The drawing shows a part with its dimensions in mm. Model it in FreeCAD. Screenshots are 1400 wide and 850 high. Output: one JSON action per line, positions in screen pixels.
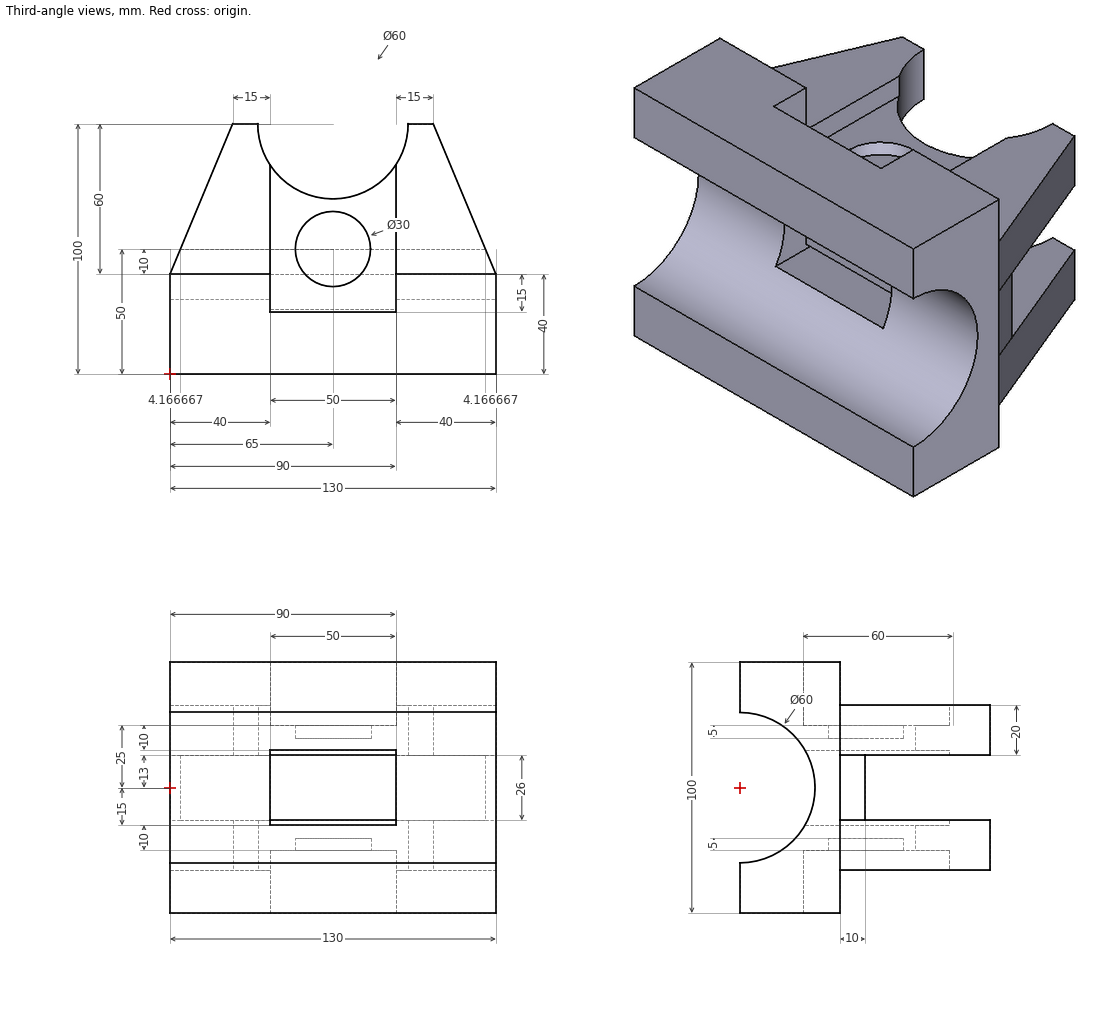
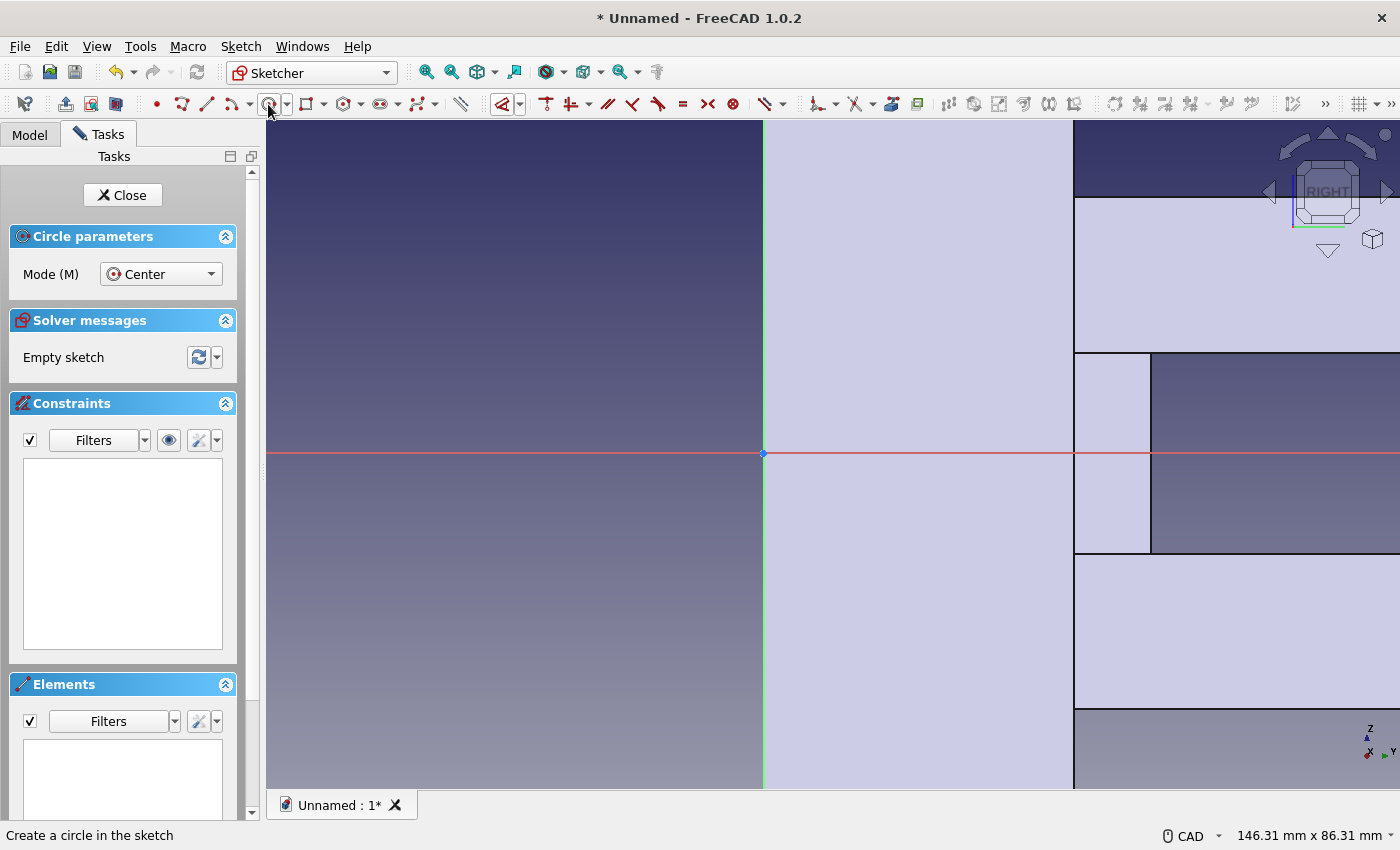
{"action": "left_click", "coordinate": [764, 453]}
{"action": "mouse_move", "coordinate": [928, 289]}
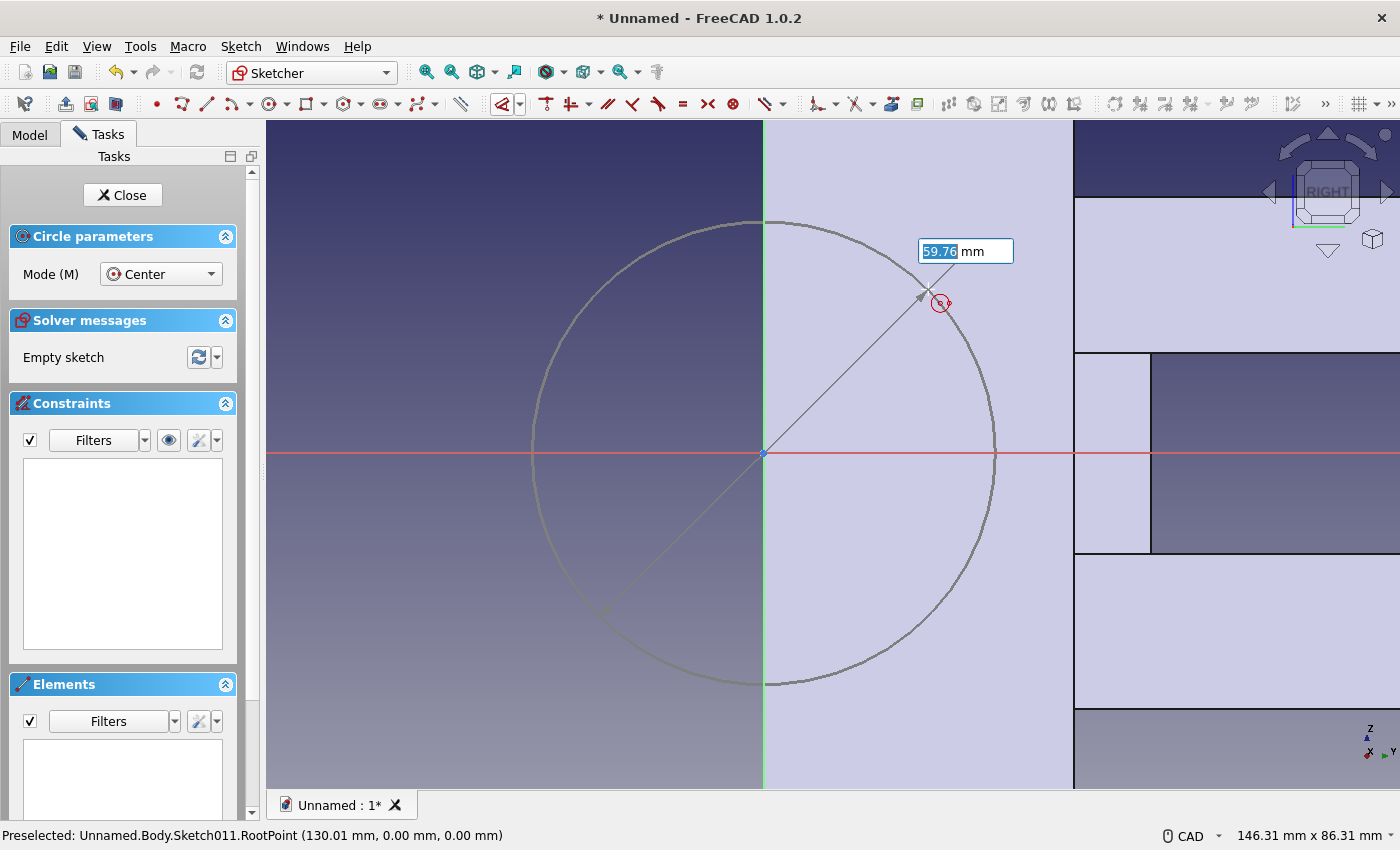
{"action": "type", "text": "60"}
{"action": "key", "text": "Return"}
{"action": "key", "text": "Escape"}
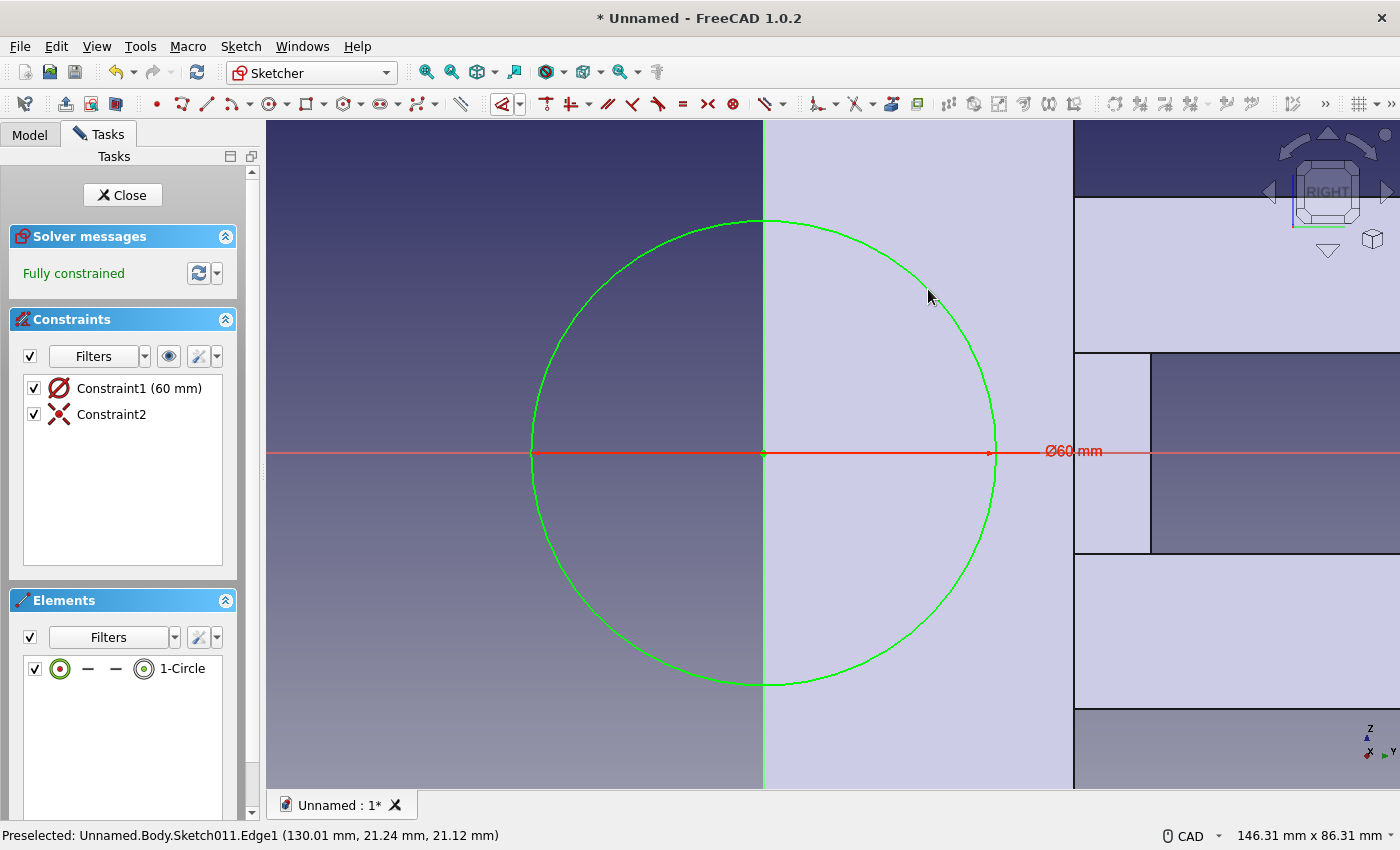
{"action": "left_click", "coordinate": [123, 195]}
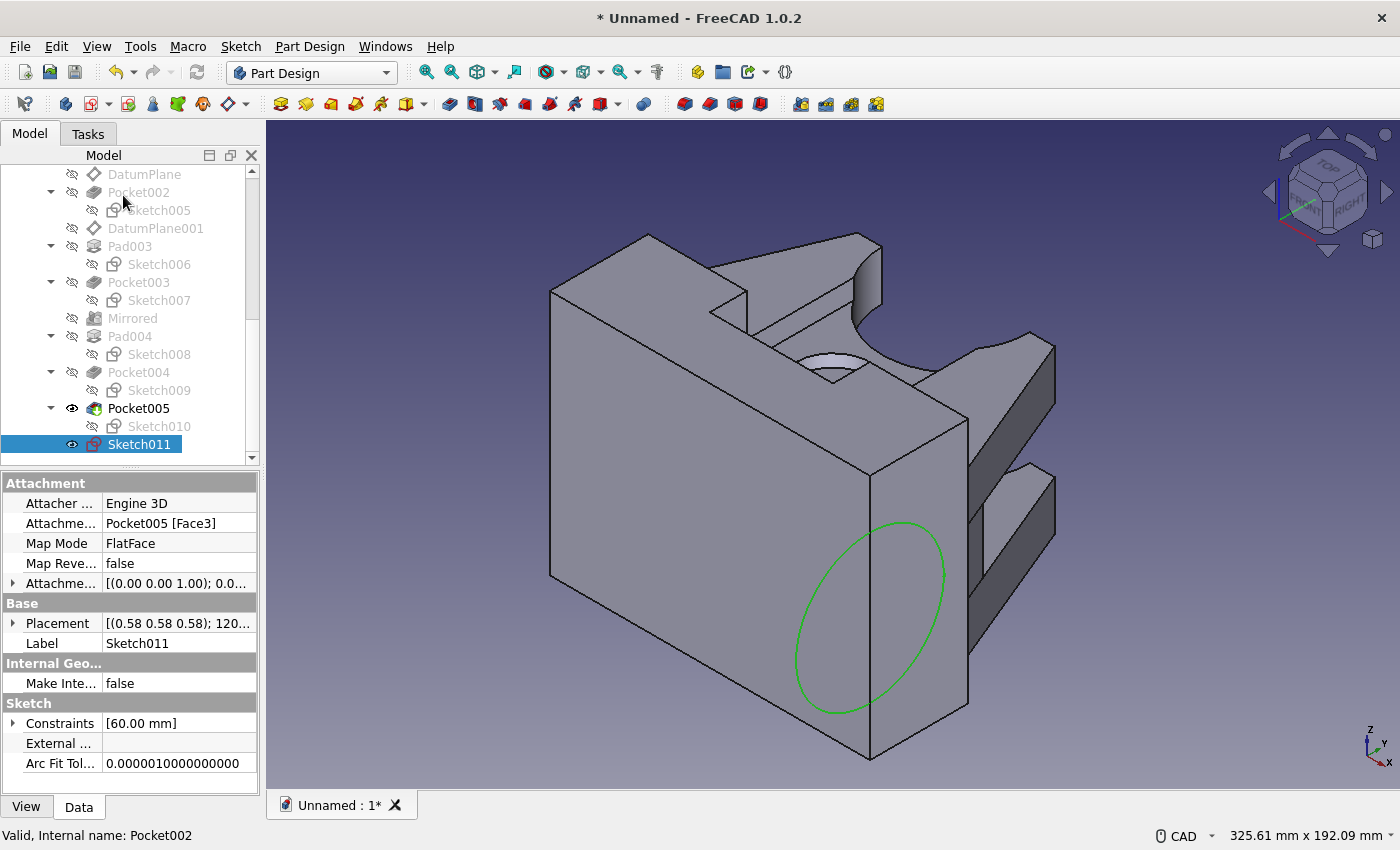
{"action": "left_click", "coordinate": [450, 104]}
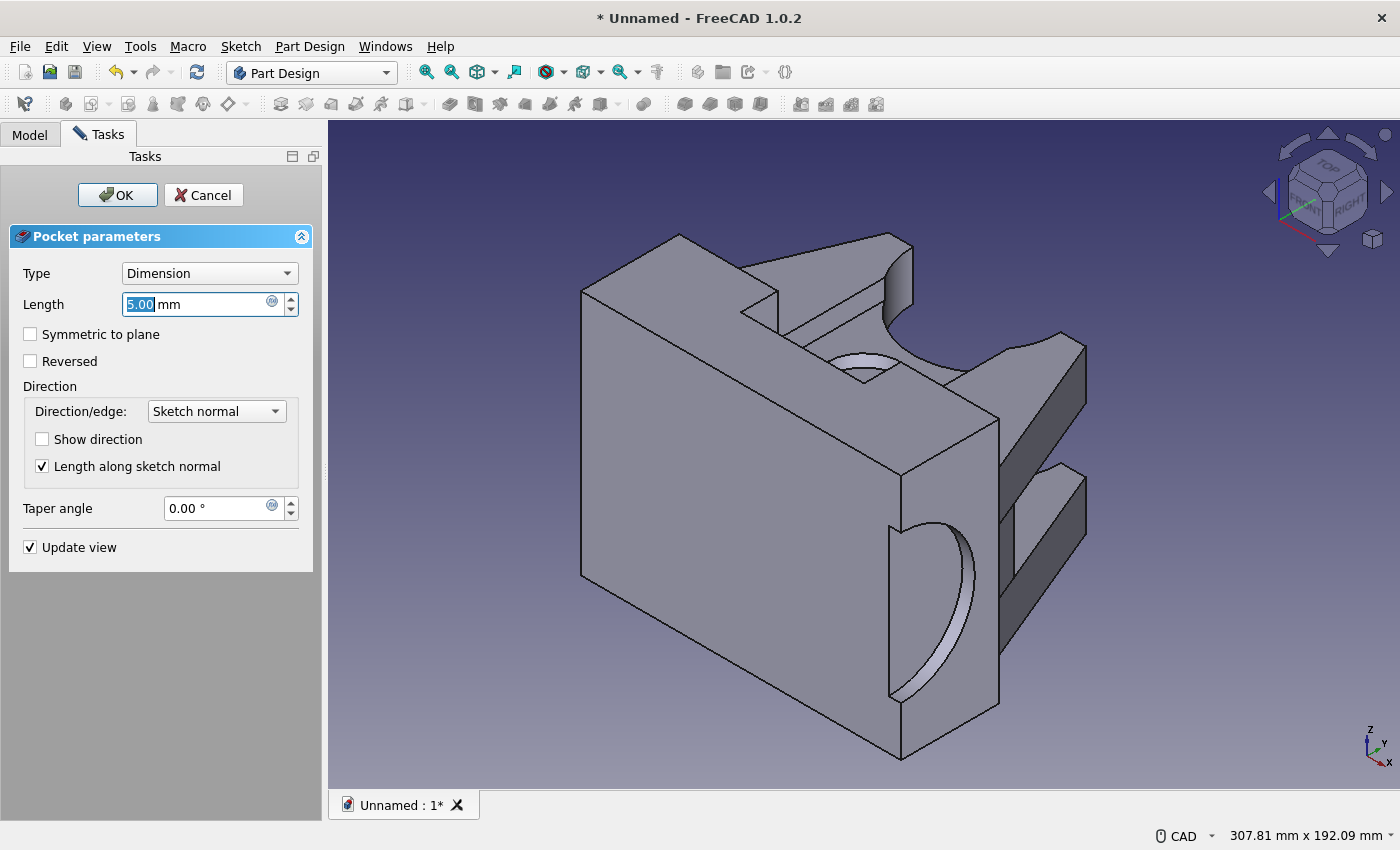
{"action": "left_click", "coordinate": [210, 274]}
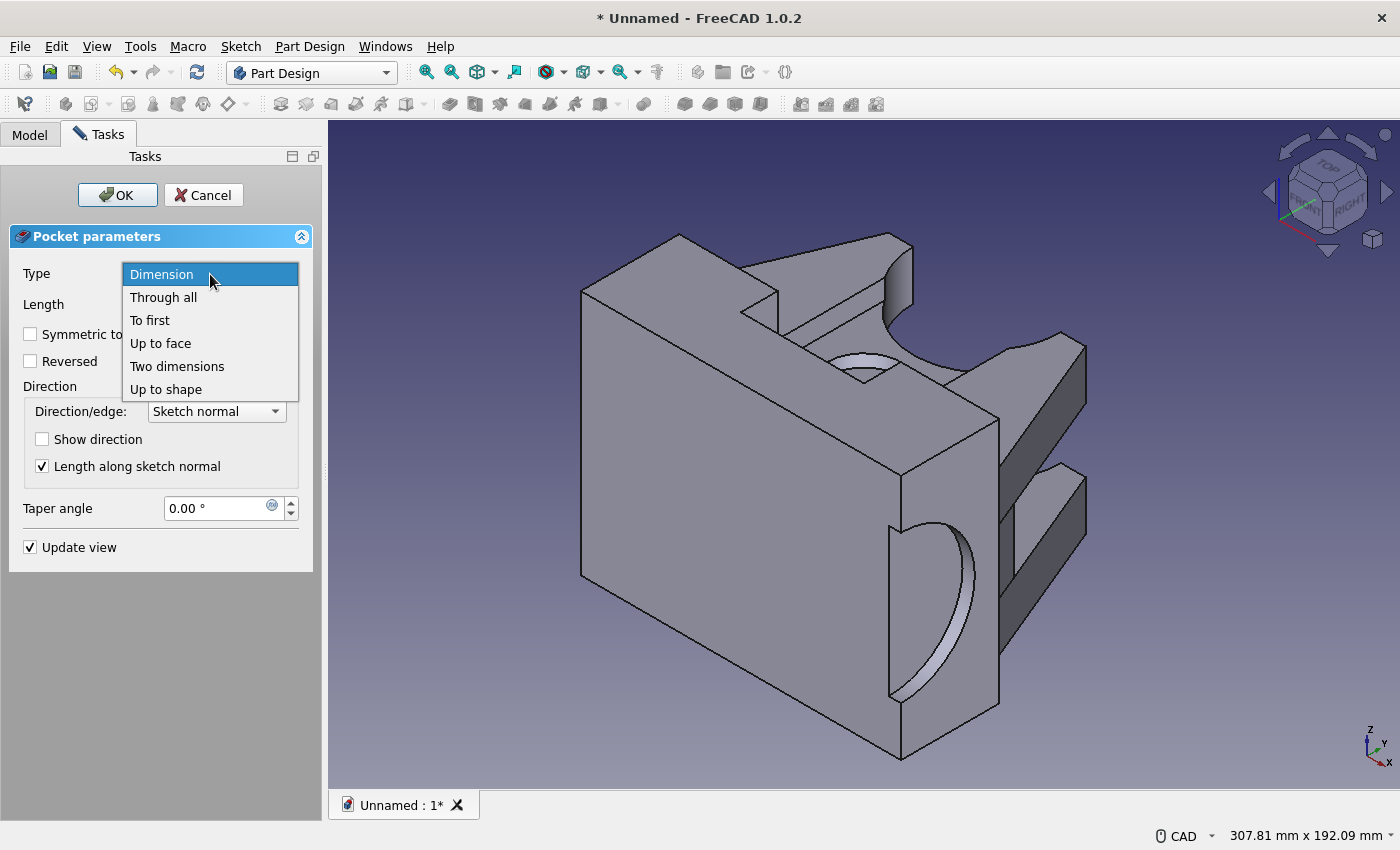
{"action": "left_click", "coordinate": [208, 298]}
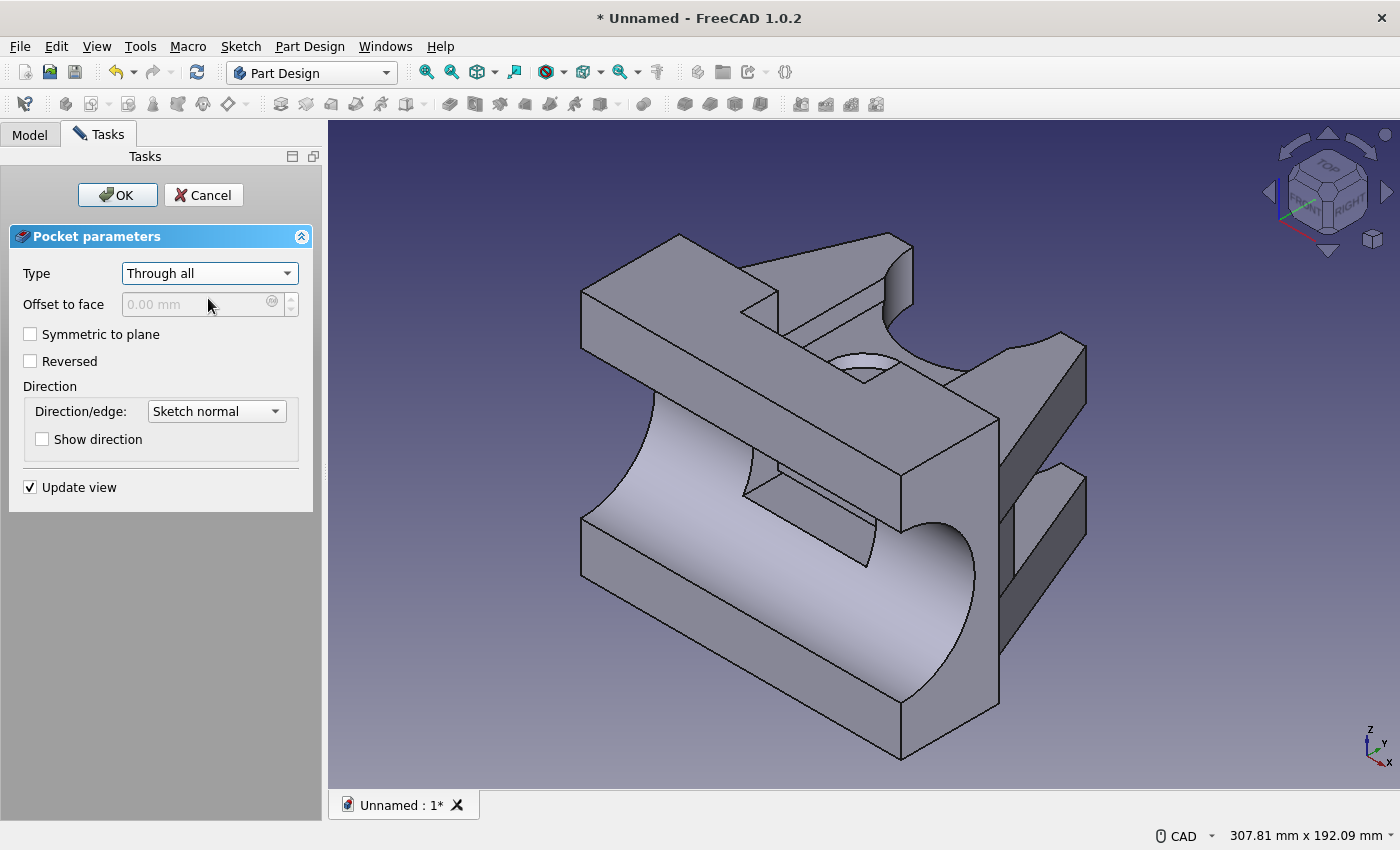
{"action": "left_click", "coordinate": [118, 195]}